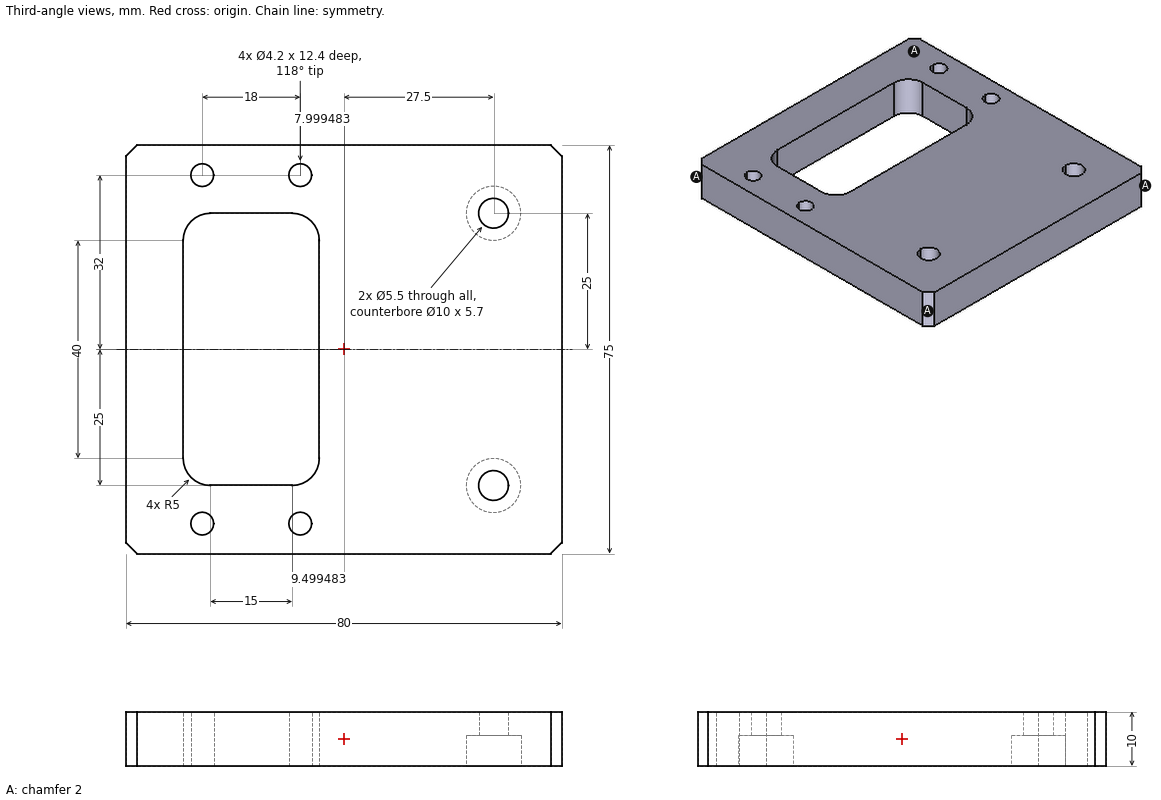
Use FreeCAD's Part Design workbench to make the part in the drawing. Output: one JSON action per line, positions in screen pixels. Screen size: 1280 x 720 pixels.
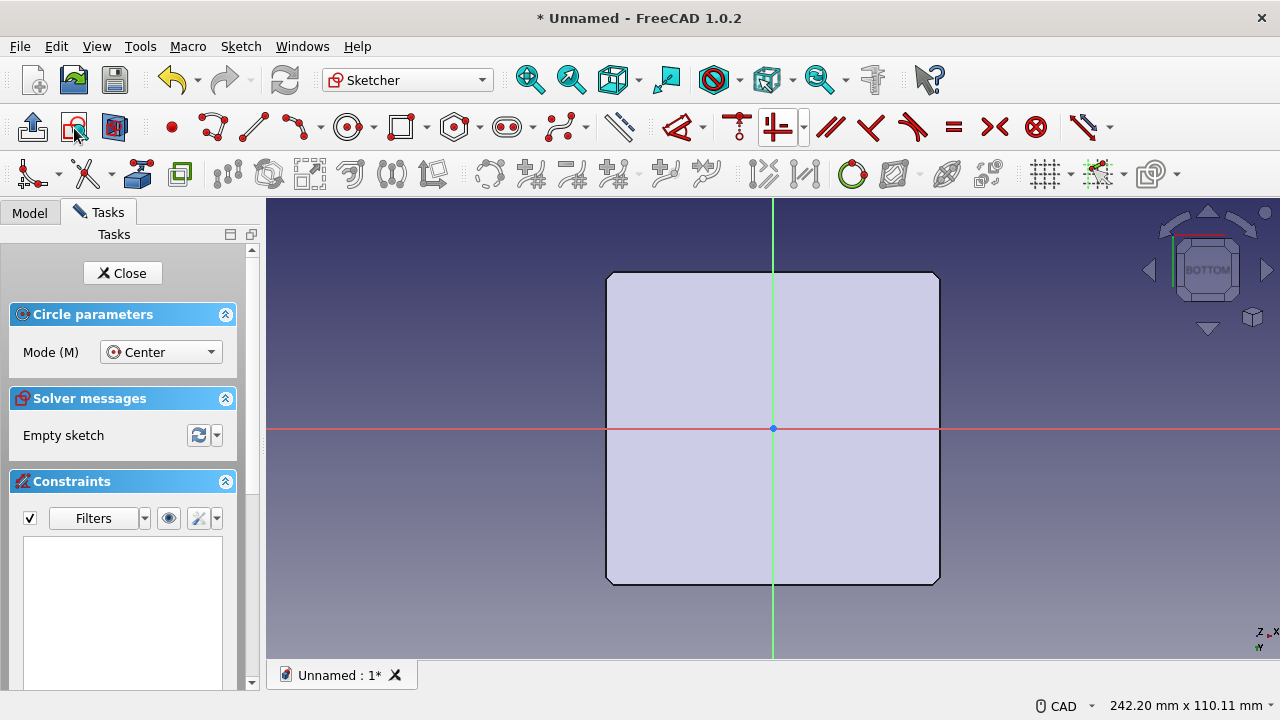
{"action": "scroll", "coordinate": [888, 533], "scroll_direction": "up", "scroll_amount": 4}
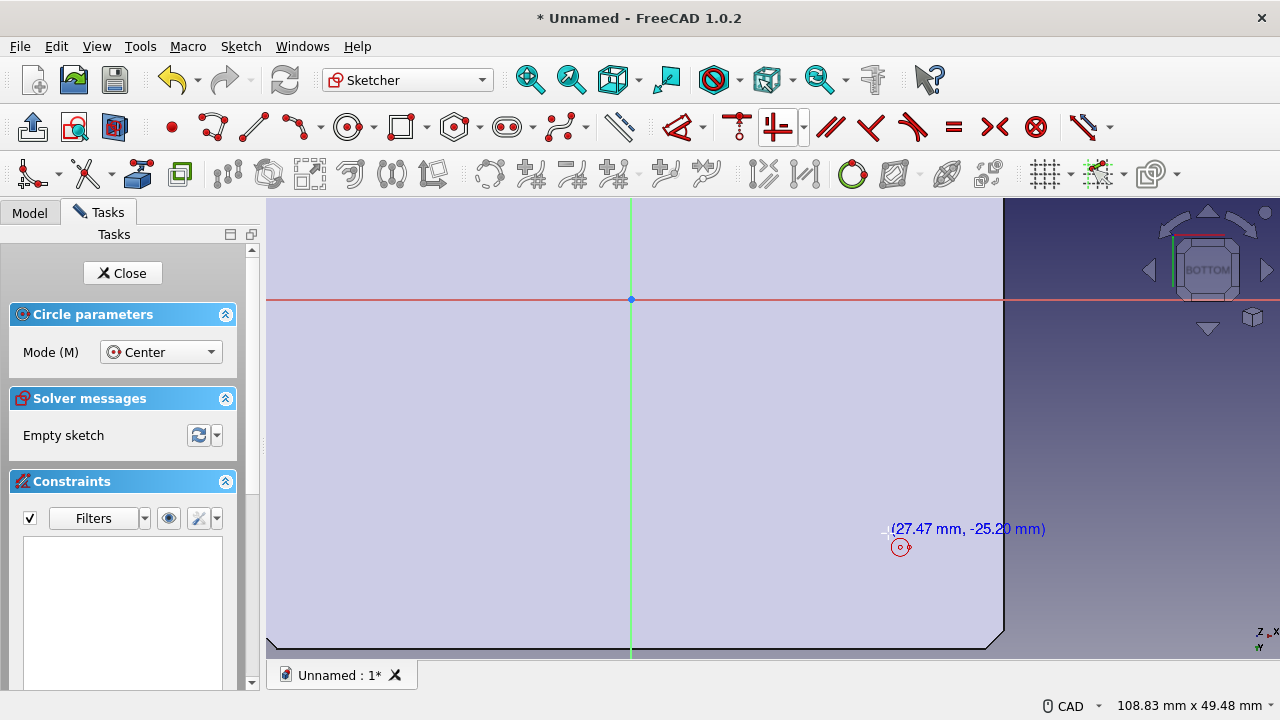
{"action": "left_click", "coordinate": [888, 532]}
{"action": "mouse_move", "coordinate": [906, 514]}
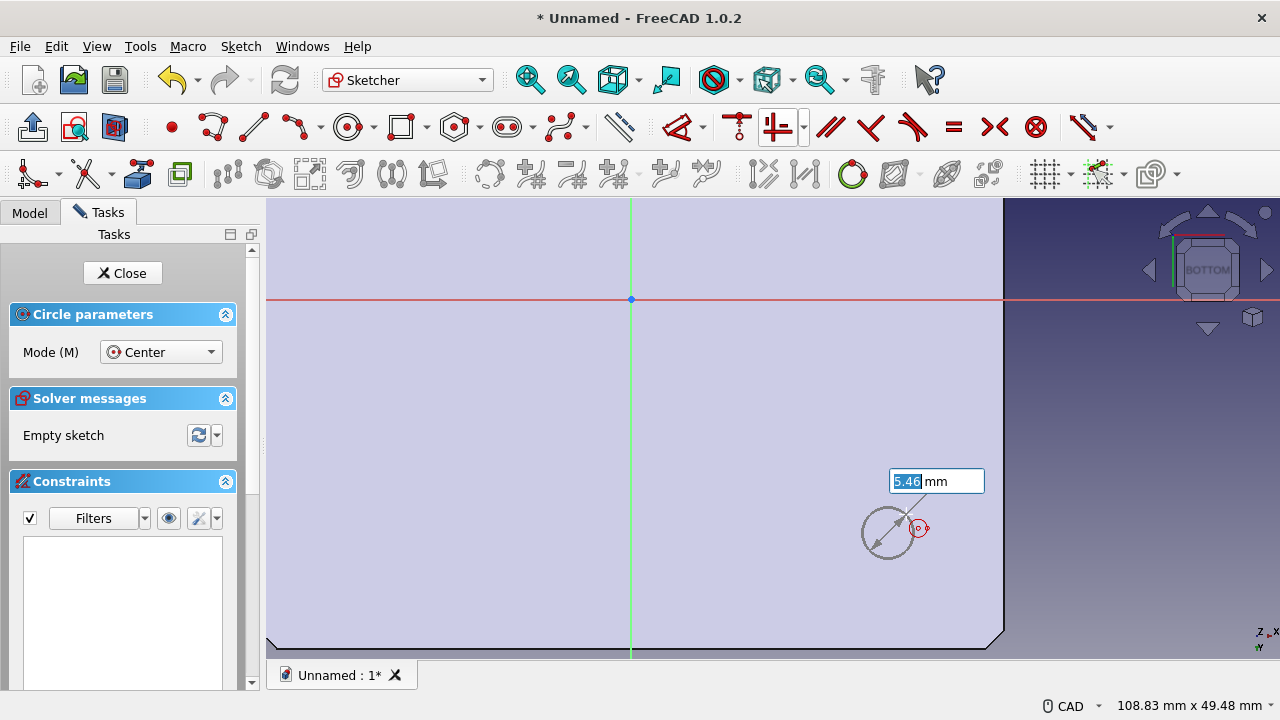
{"action": "type", "text": "5.5"}
{"action": "key", "text": "Return"}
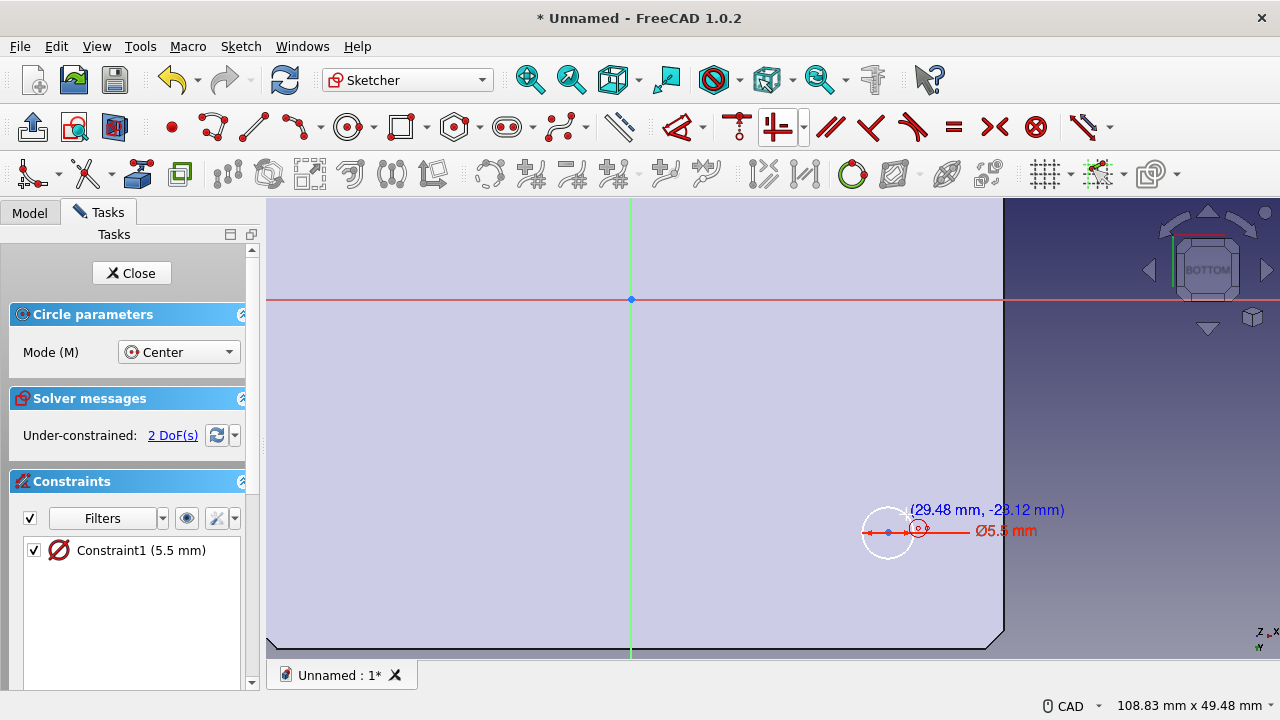
{"action": "scroll", "coordinate": [622, 585], "scroll_direction": "down", "scroll_amount": 3}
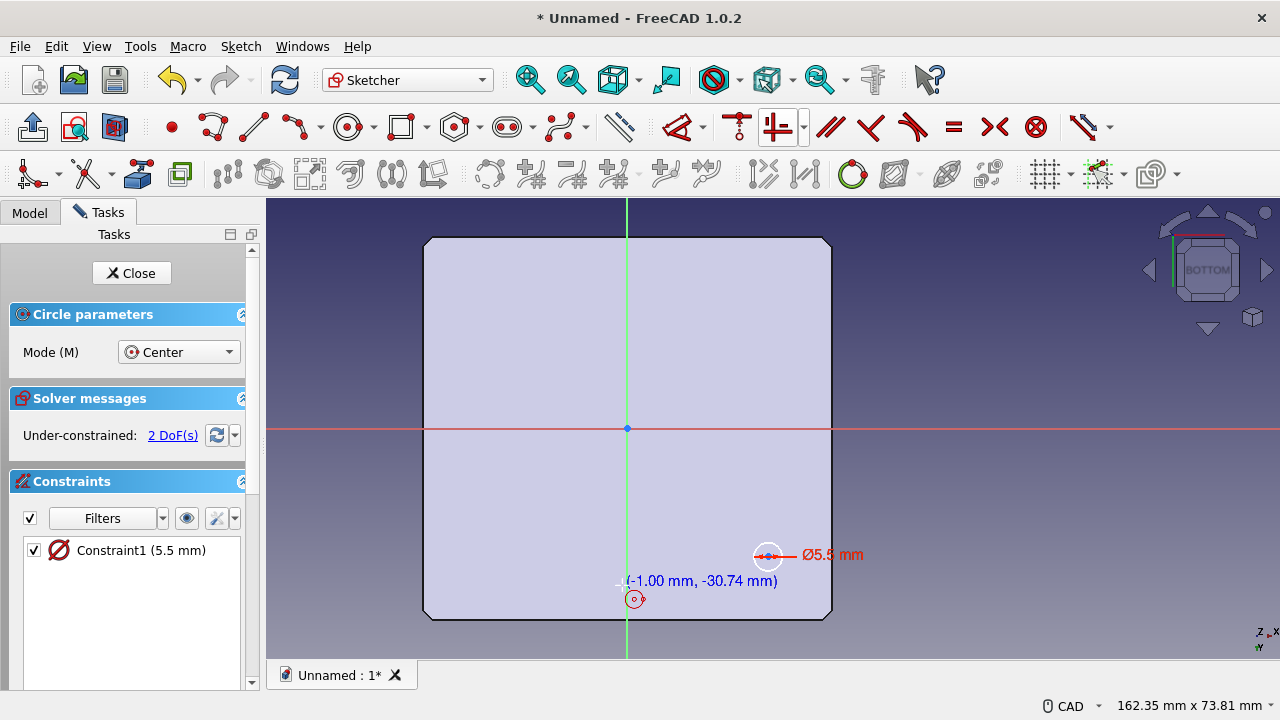
{"action": "scroll", "coordinate": [768, 301], "scroll_direction": "up", "scroll_amount": 3}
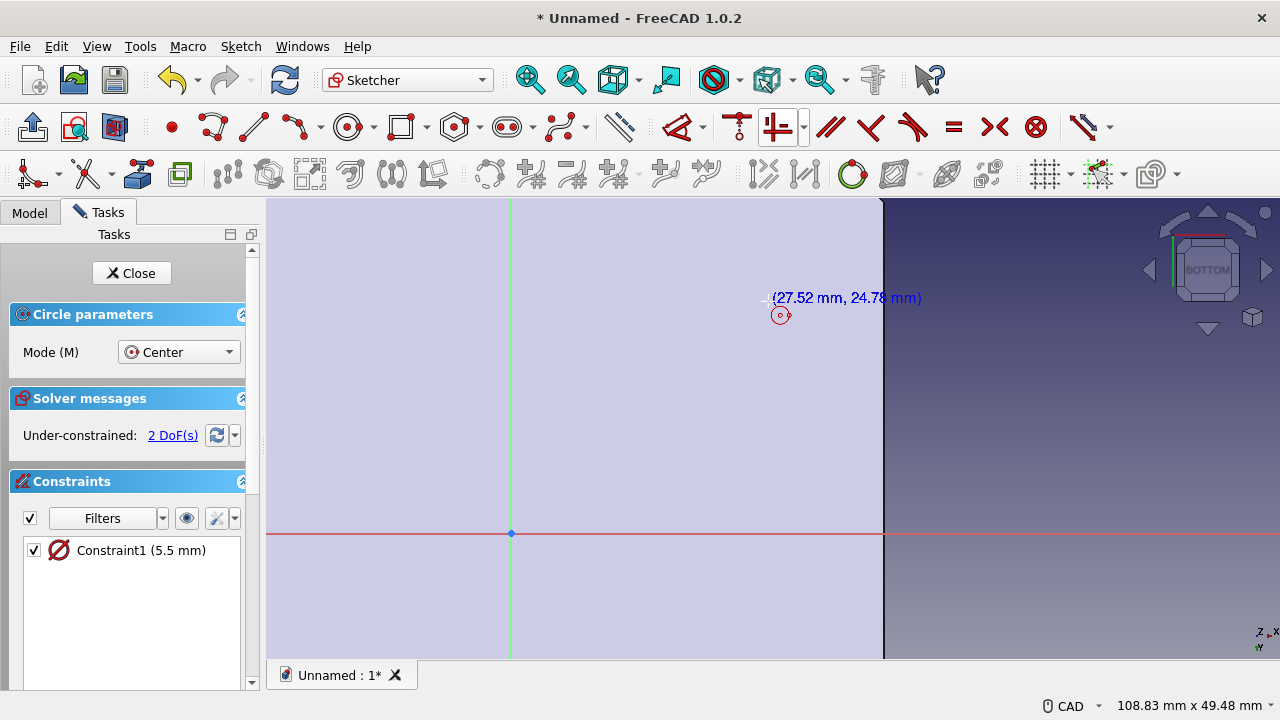
{"action": "left_click", "coordinate": [767, 301]}
{"action": "mouse_move", "coordinate": [786, 282]}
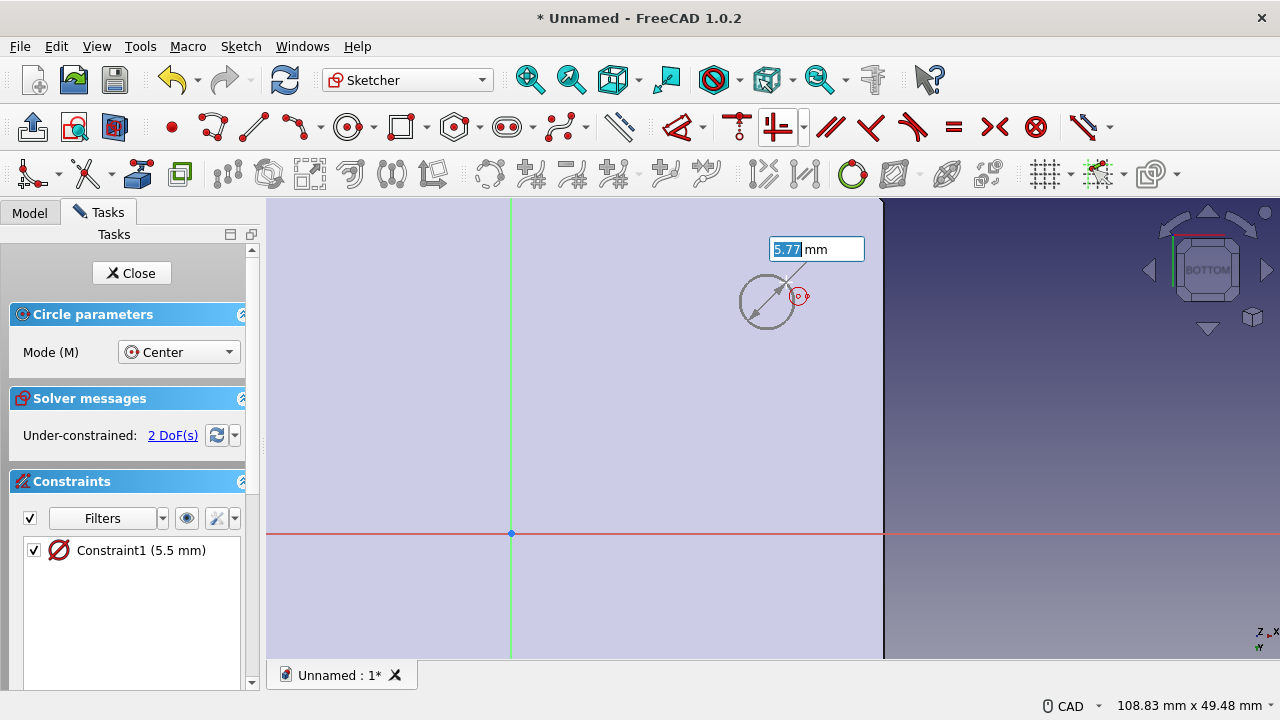
{"action": "type", "text": "5.5"}
{"action": "key", "text": "Return"}
{"action": "key", "text": "Escape"}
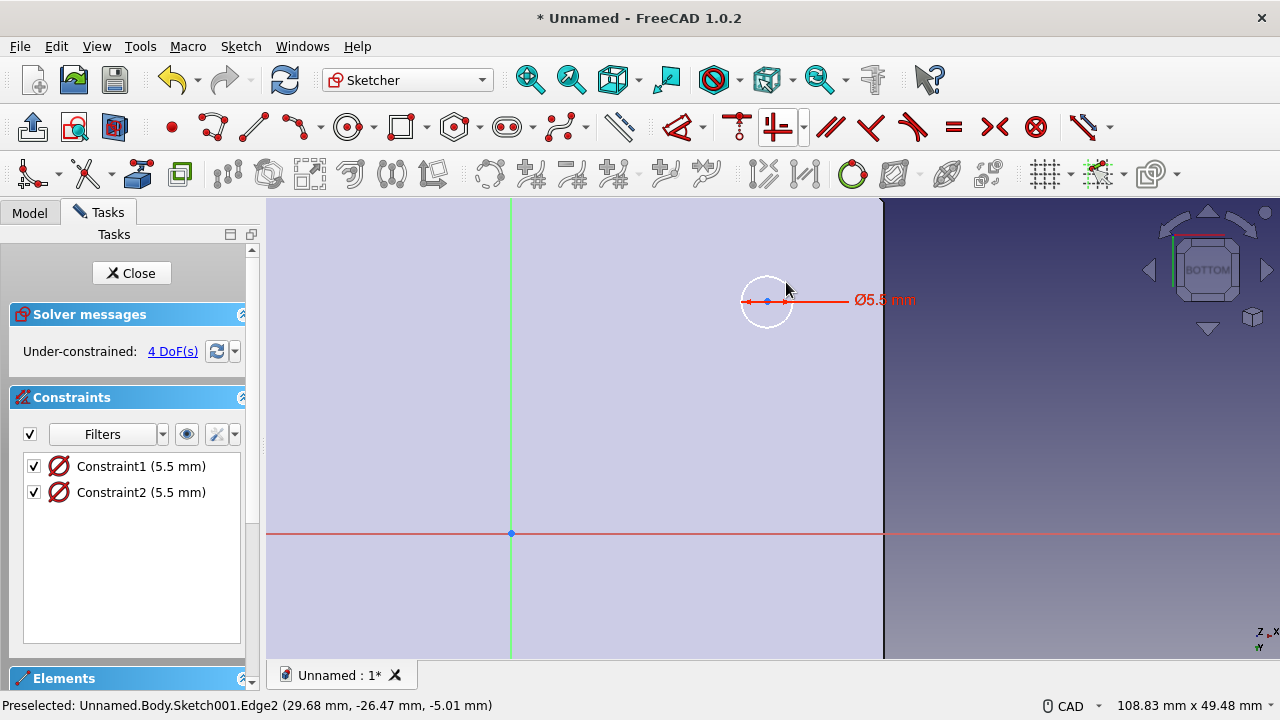
{"action": "scroll", "coordinate": [768, 301], "scroll_direction": "down", "scroll_amount": 3}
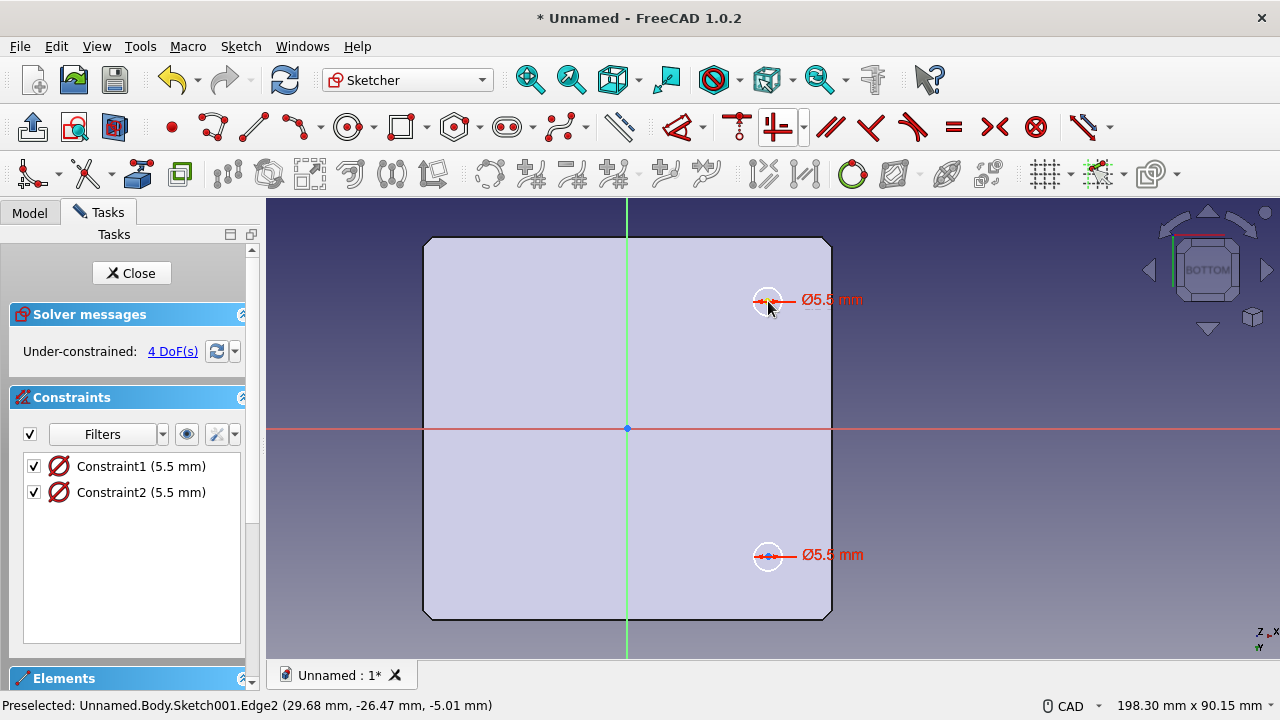
{"action": "left_click", "coordinate": [768, 557]}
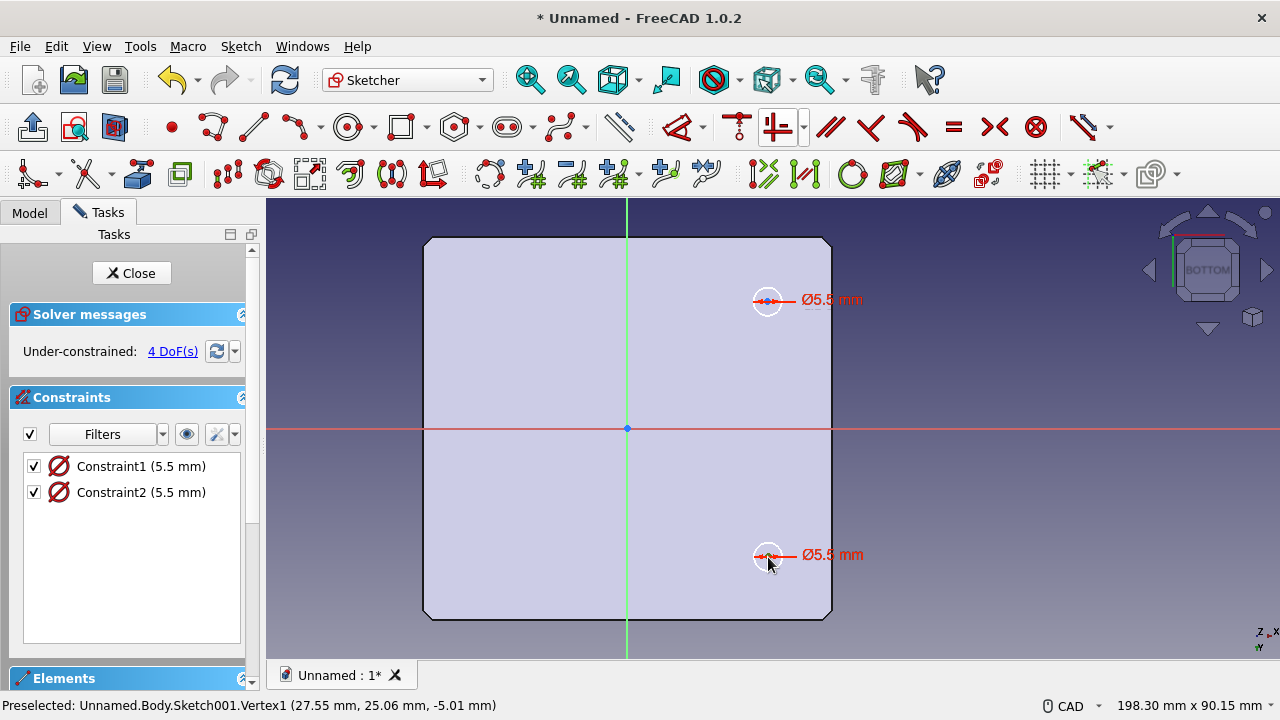
{"action": "left_click", "coordinate": [768, 302]}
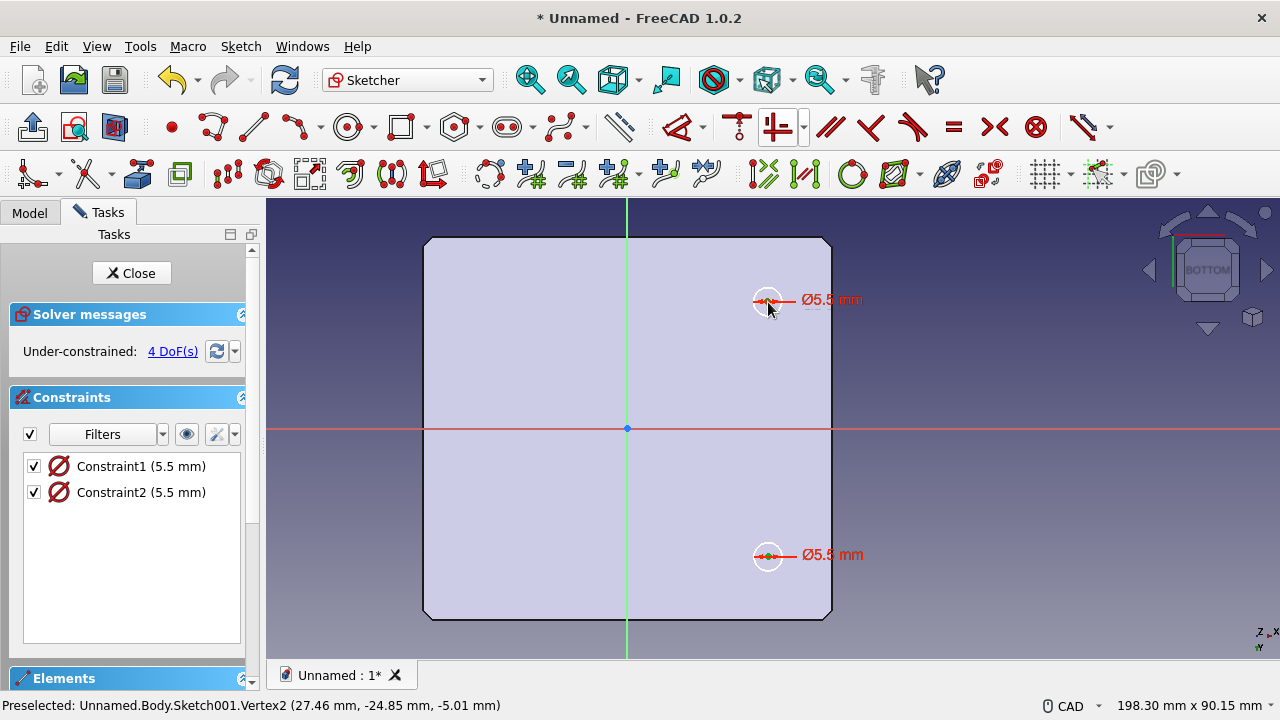
{"action": "left_click", "coordinate": [353, 429]}